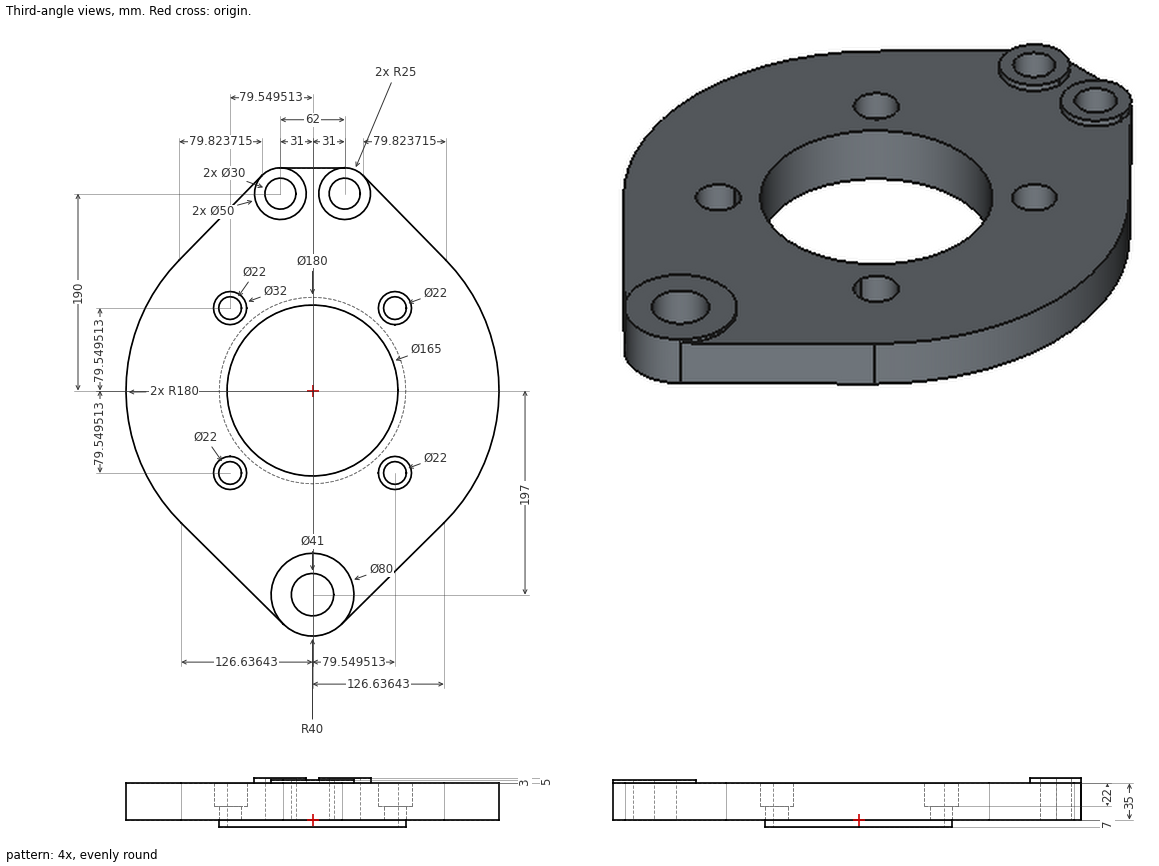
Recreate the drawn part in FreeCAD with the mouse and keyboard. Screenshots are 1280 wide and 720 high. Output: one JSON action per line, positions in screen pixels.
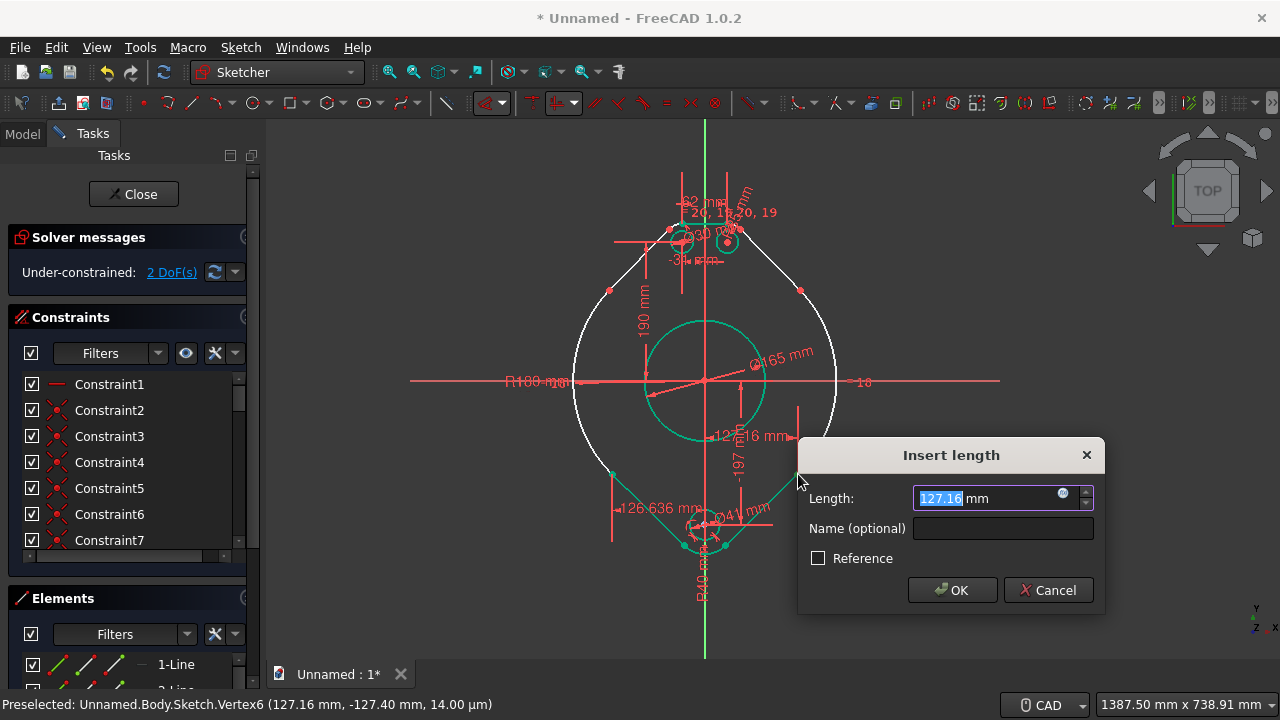
{"action": "type", "text": "126.63643"}
{"action": "key", "text": "Return"}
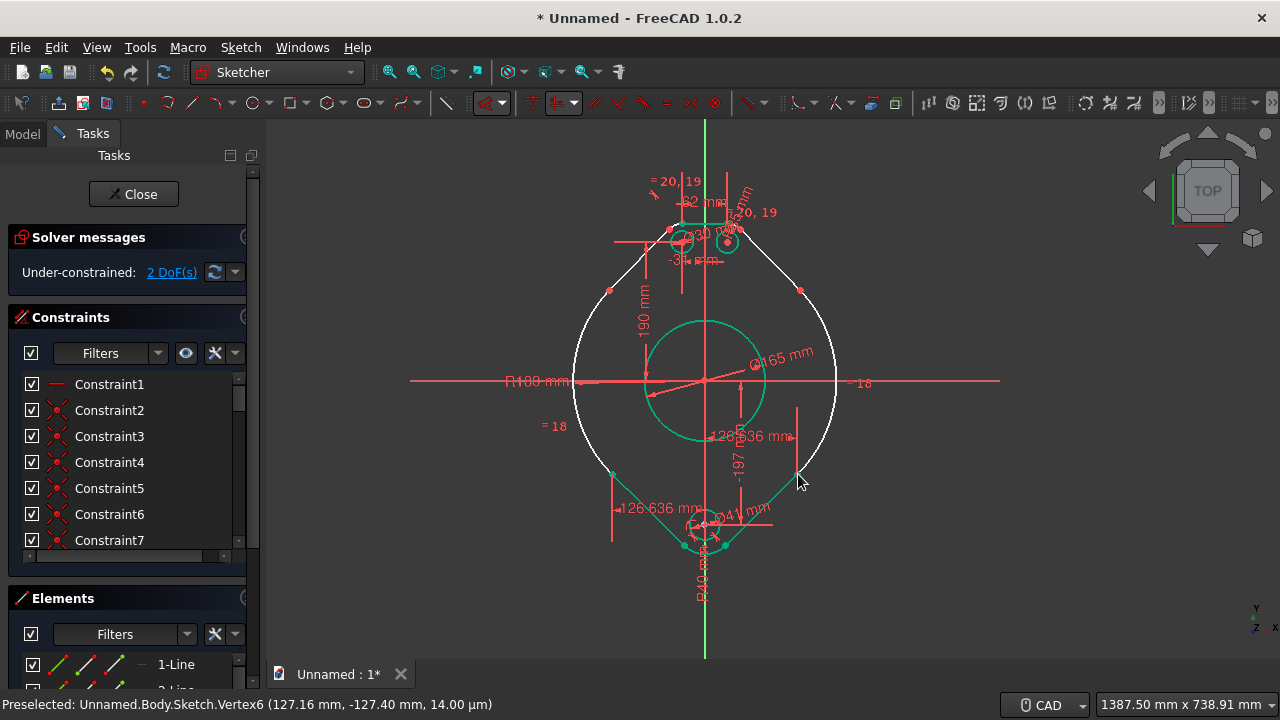
{"action": "left_click", "coordinate": [651, 248]}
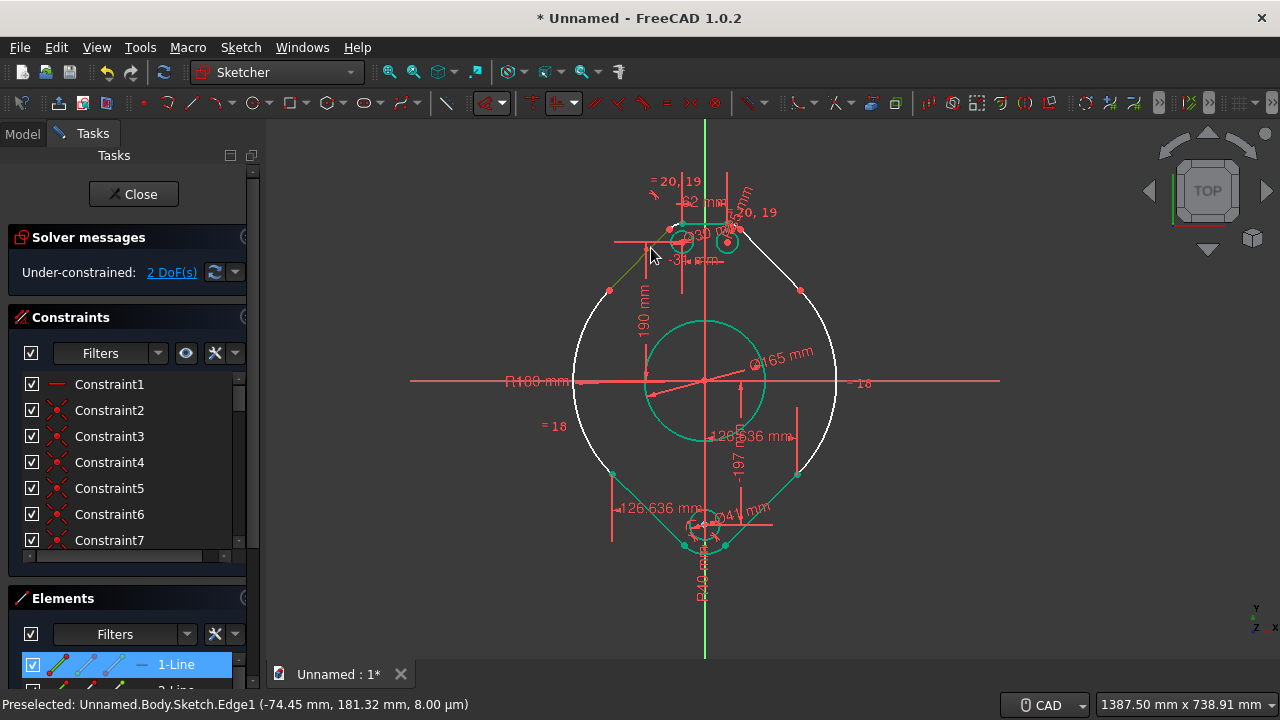
{"action": "key", "text": "l"}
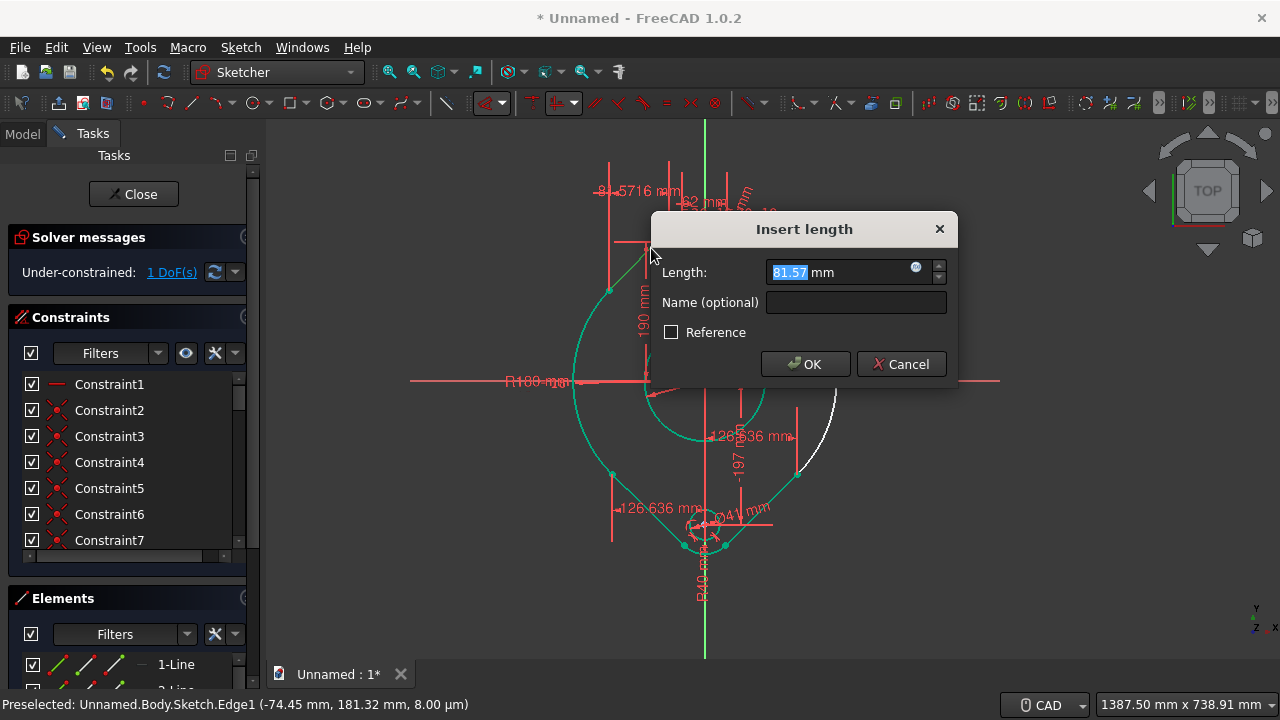
{"action": "type", "text": "79.823715"}
{"action": "key", "text": "Return"}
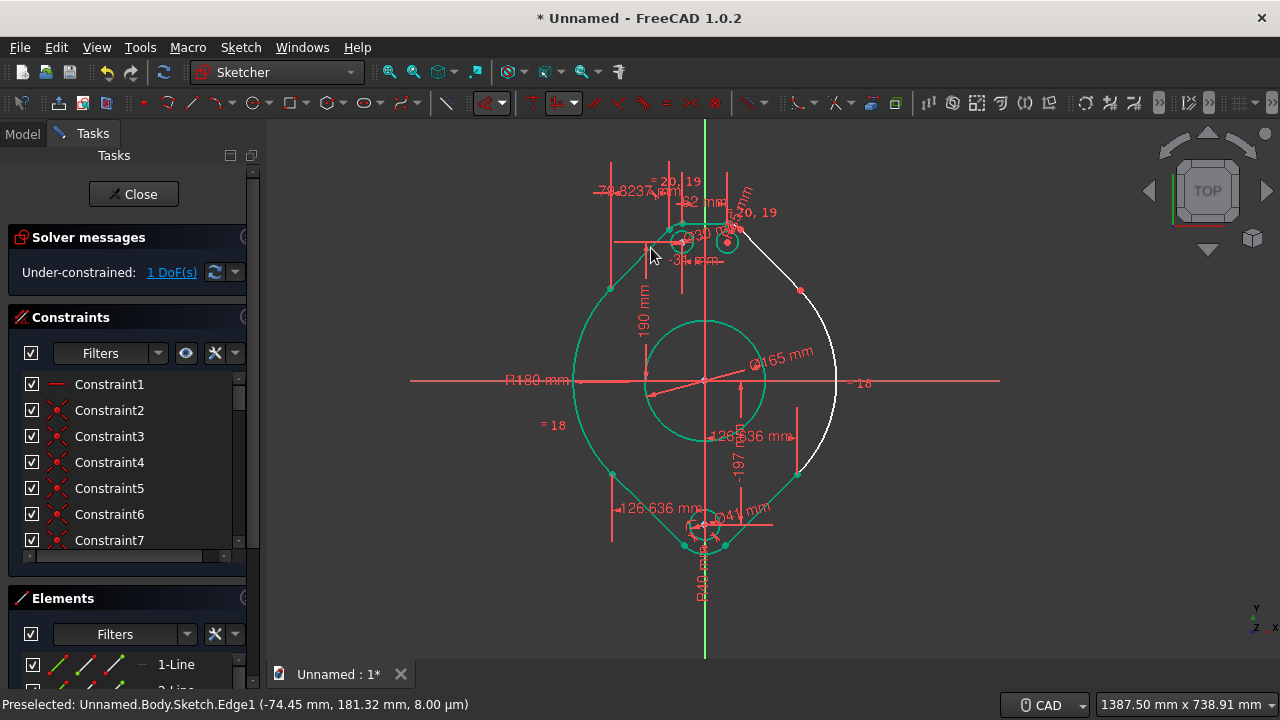
{"action": "left_click", "coordinate": [782, 272]}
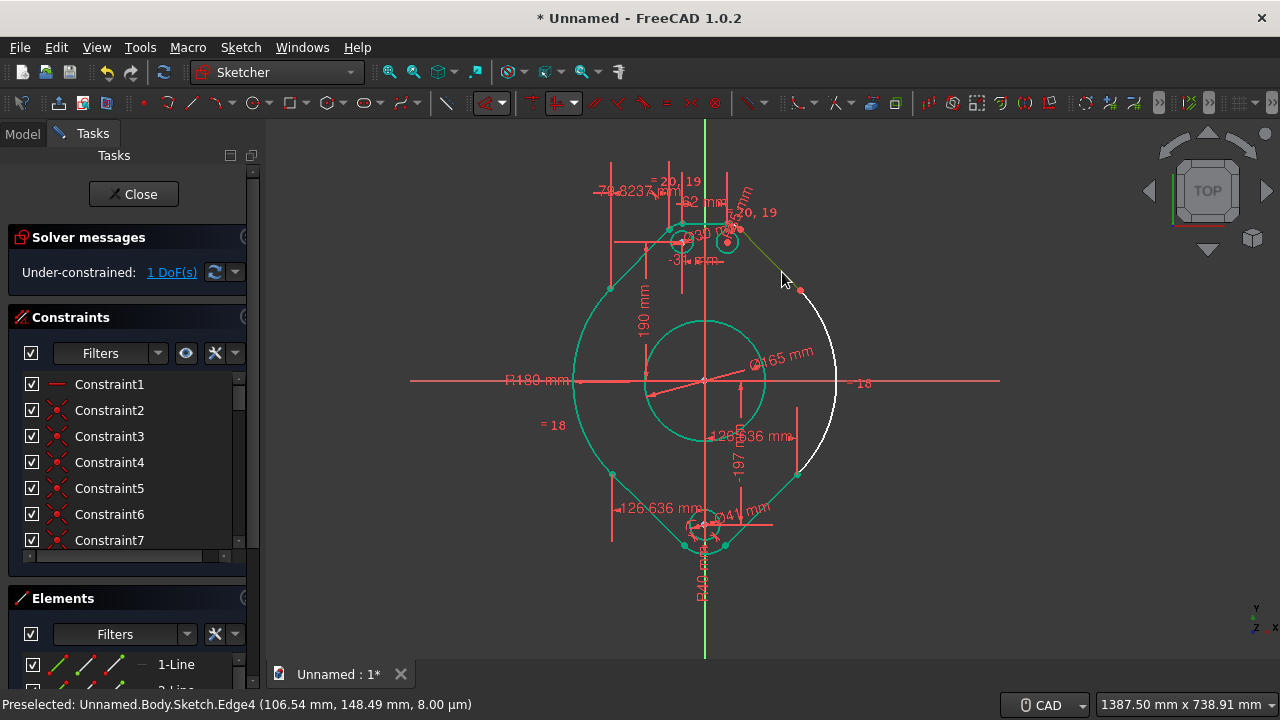
{"action": "key", "text": "l"}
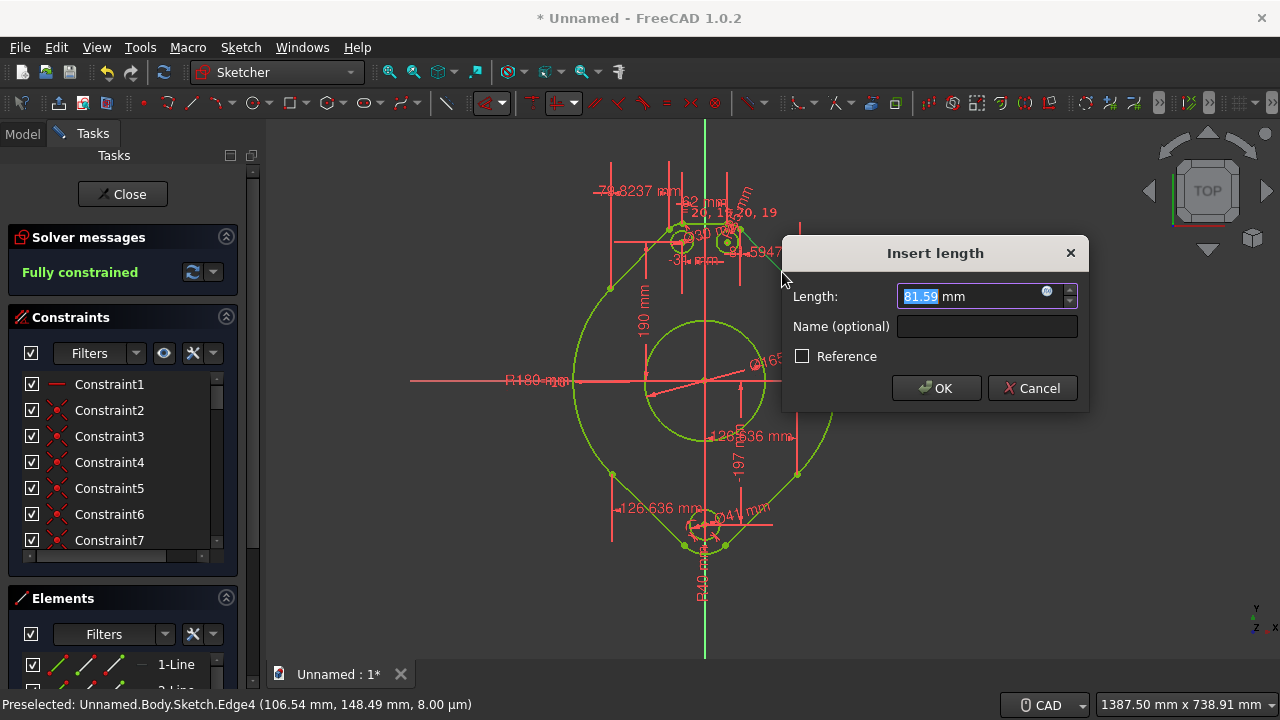
{"action": "type", "text": "79.823715"}
{"action": "key", "text": "Return"}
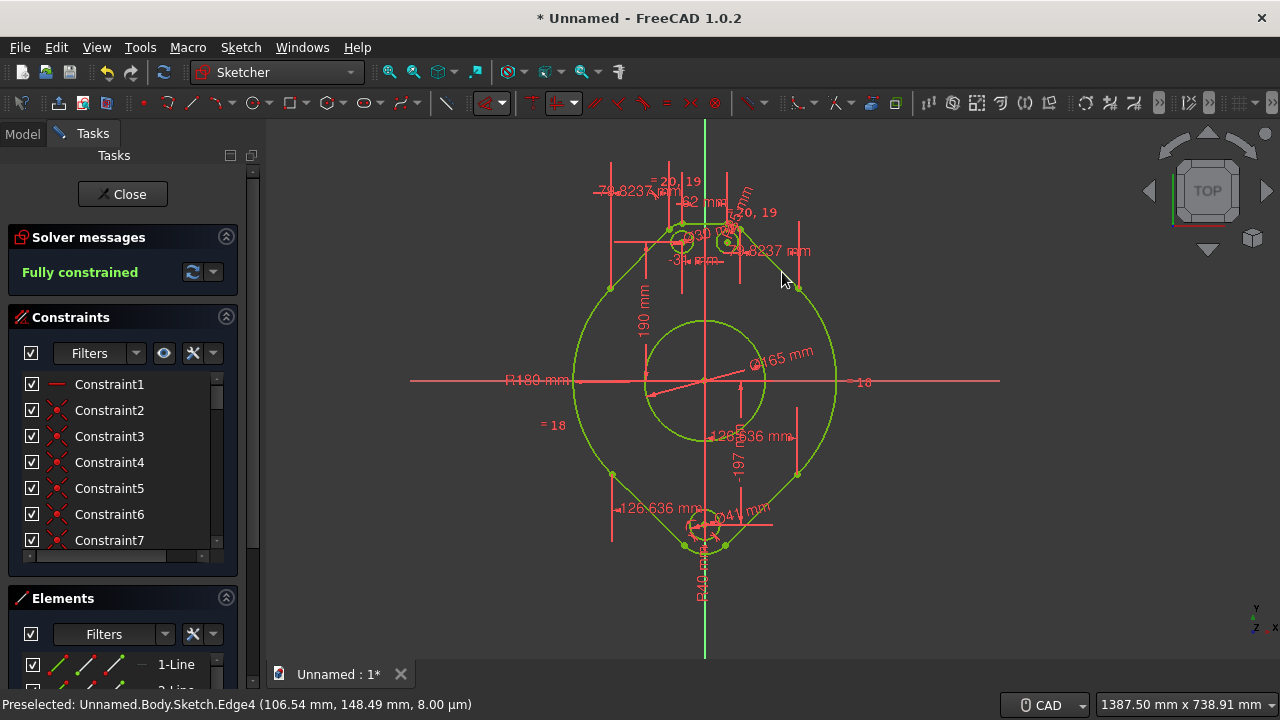
{"action": "left_click", "coordinate": [123, 194]}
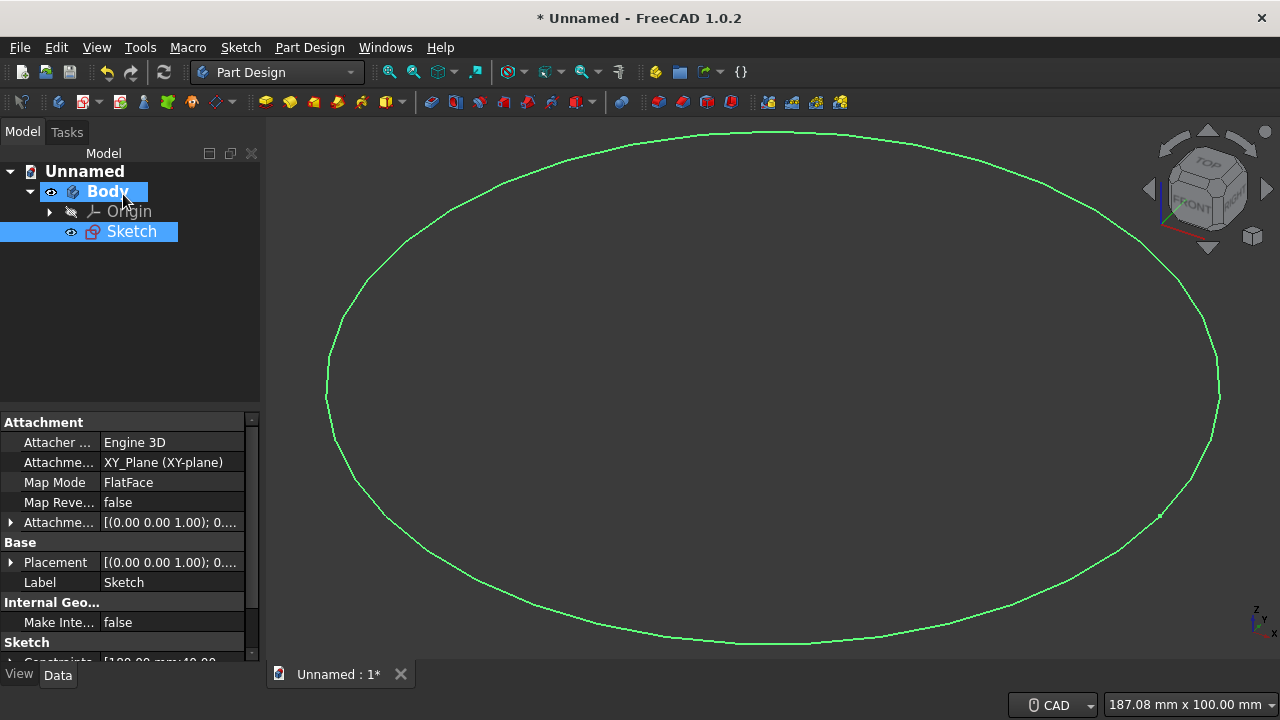
{"action": "left_click", "coordinate": [266, 102]}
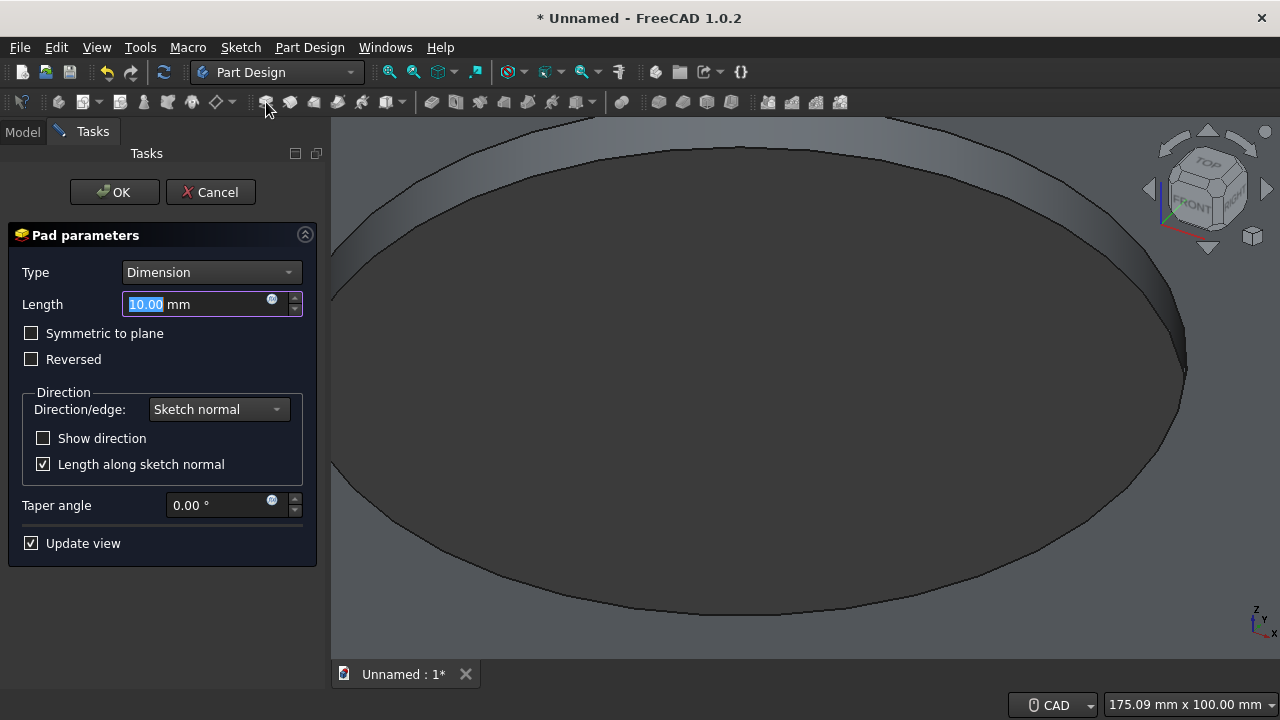
{"action": "type", "text": "35"}
{"action": "key", "text": "Tab"}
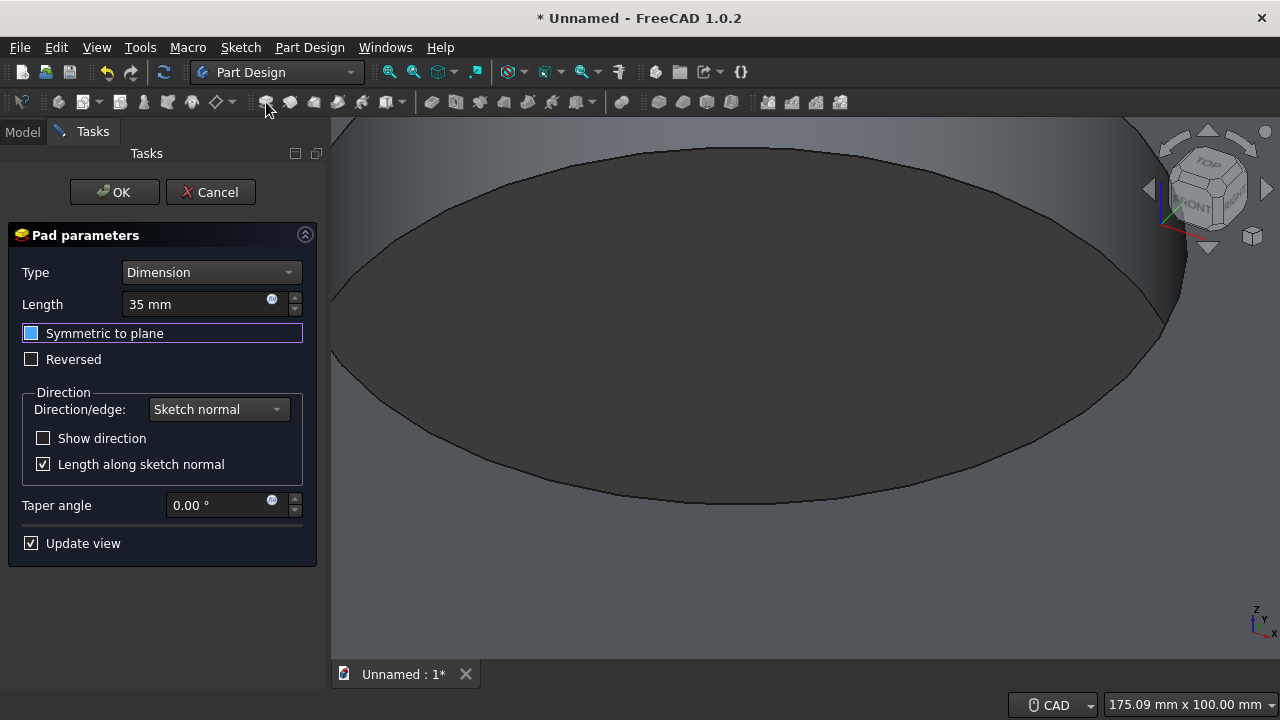
{"action": "left_click", "coordinate": [115, 192]}